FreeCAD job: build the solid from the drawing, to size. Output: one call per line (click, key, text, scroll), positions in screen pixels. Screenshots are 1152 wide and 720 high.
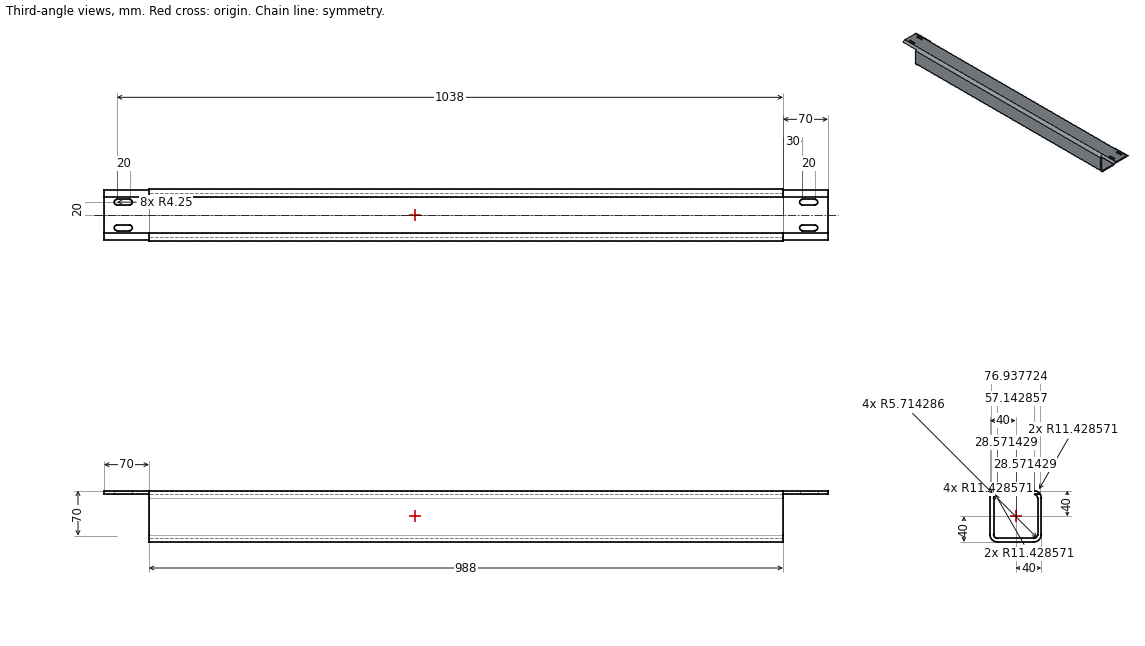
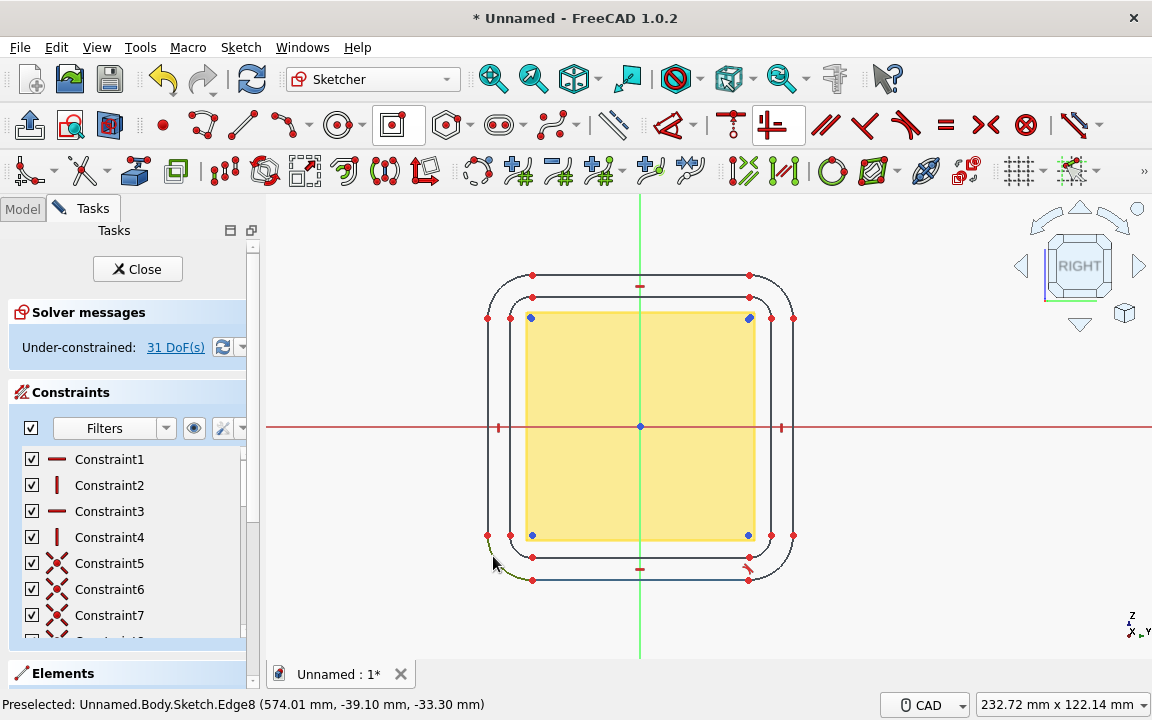
click(906, 126)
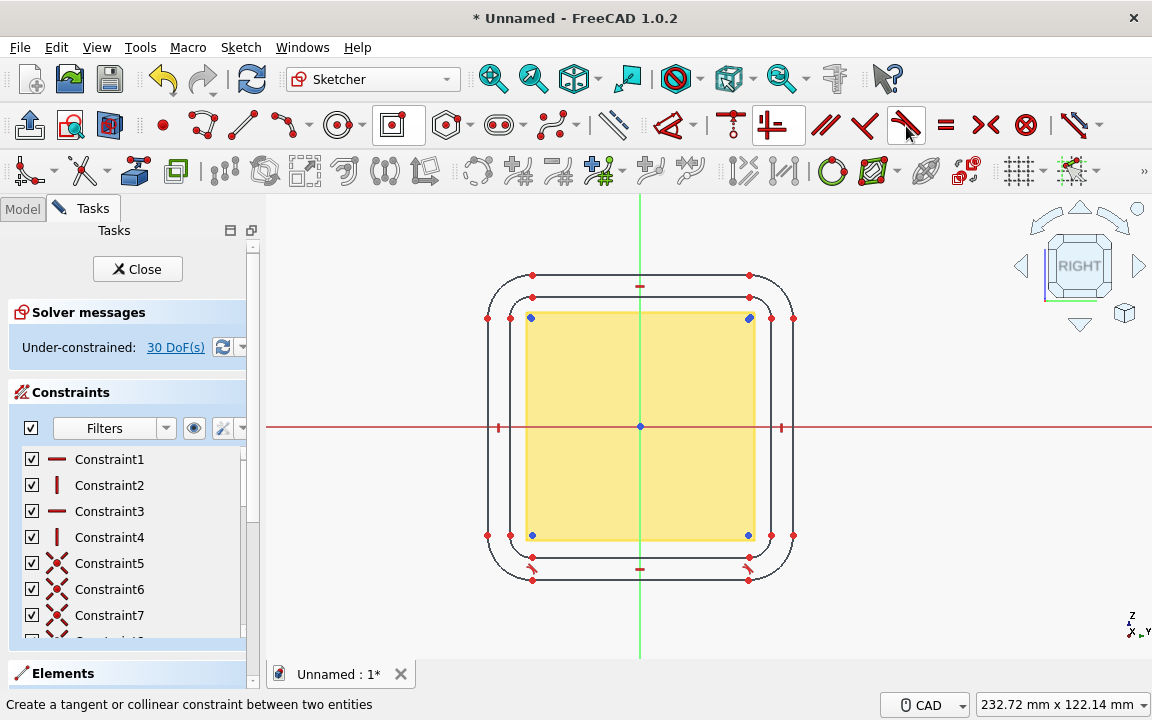
click(793, 471)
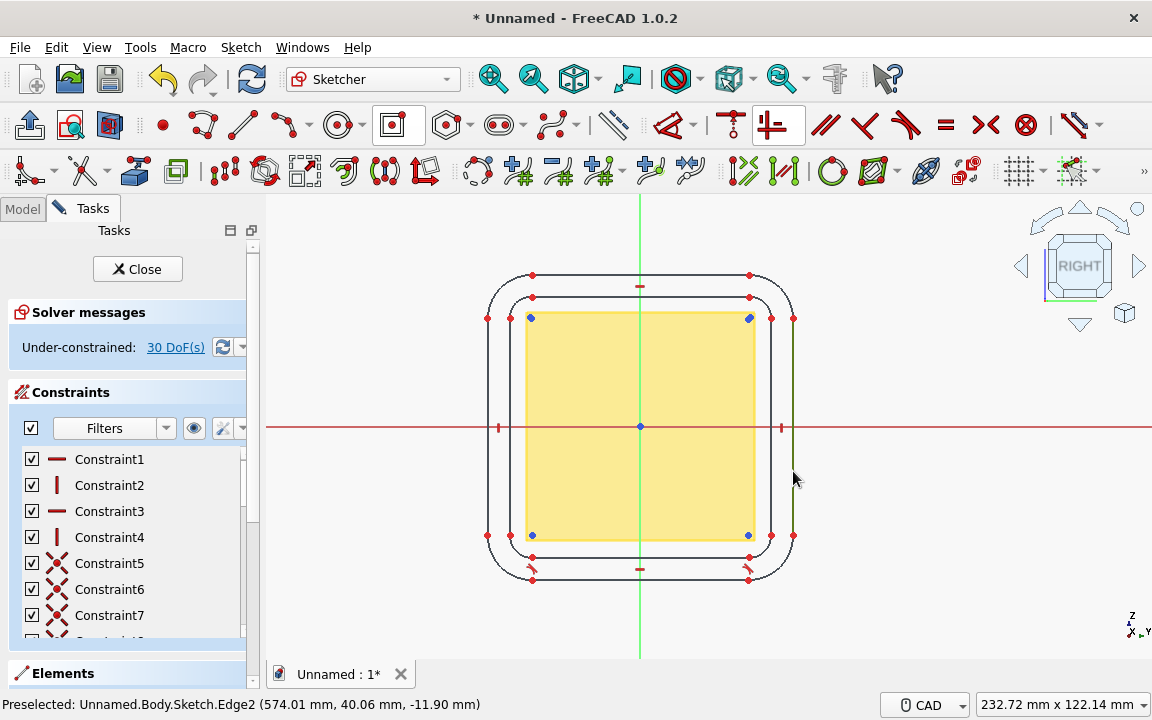
click(769, 575)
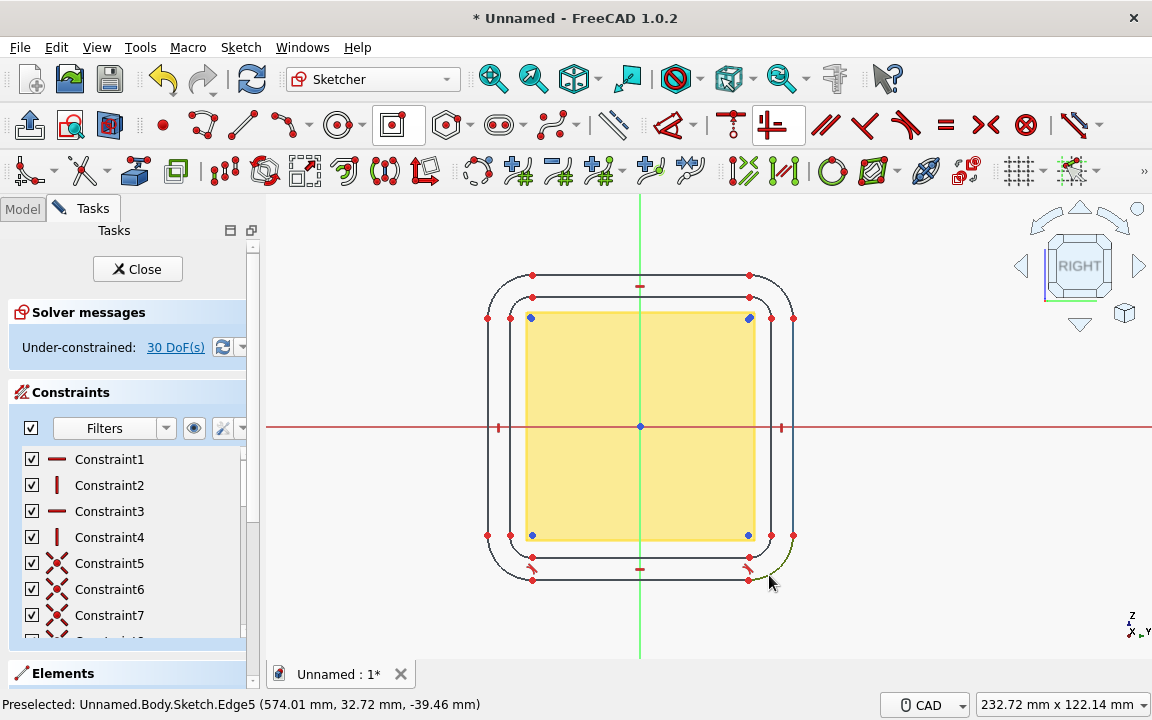
key(t)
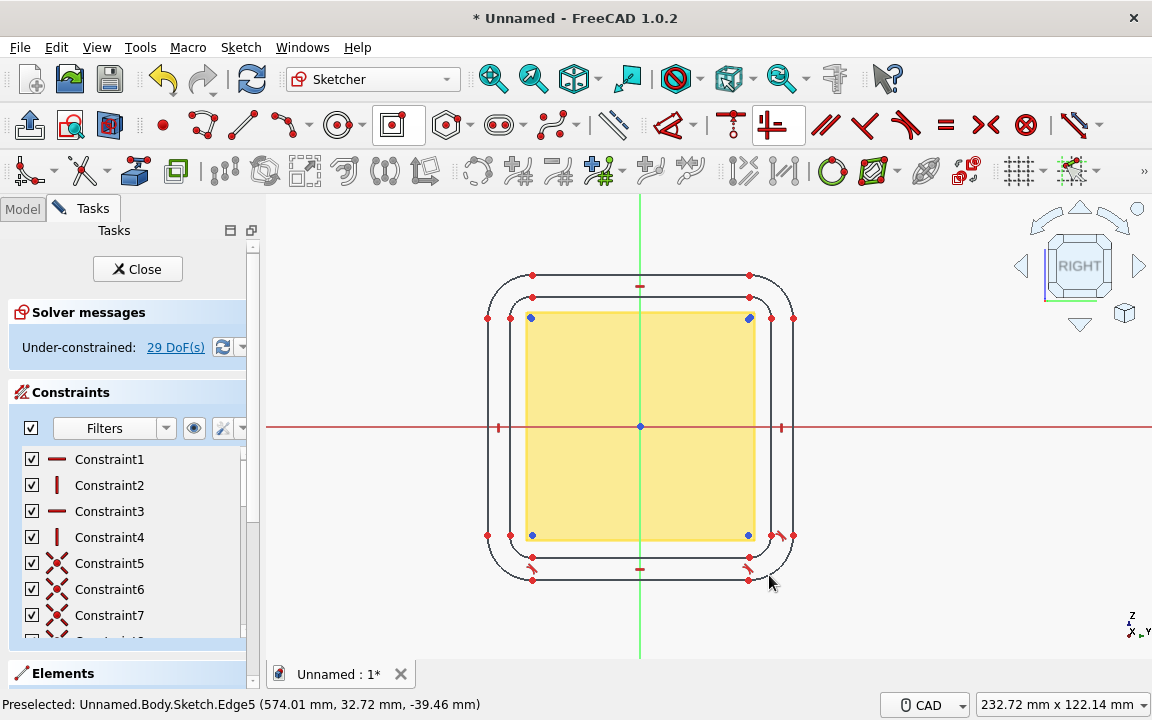
click(793, 471)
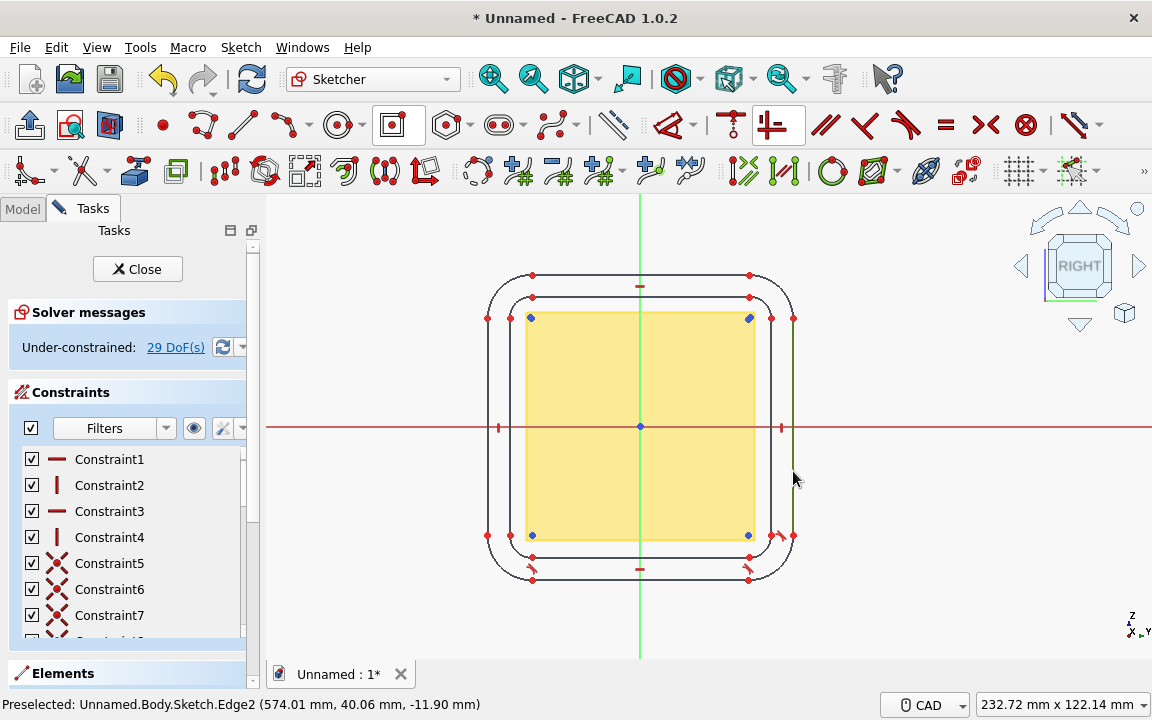
click(788, 299)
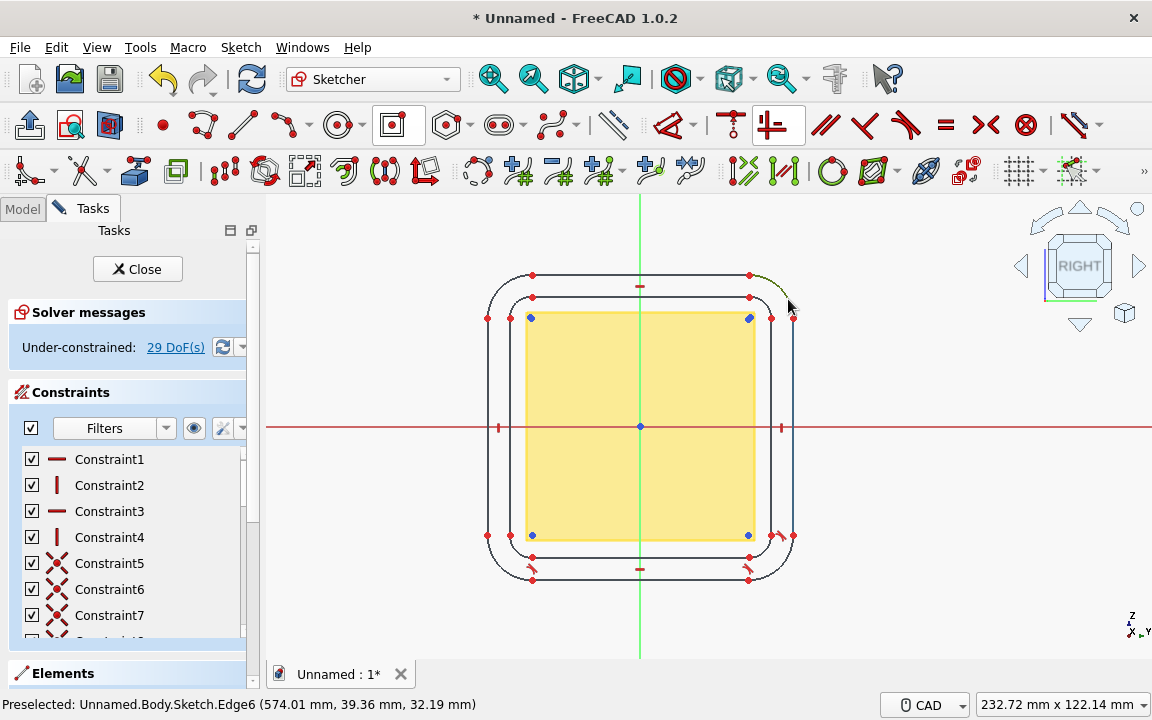
key(t)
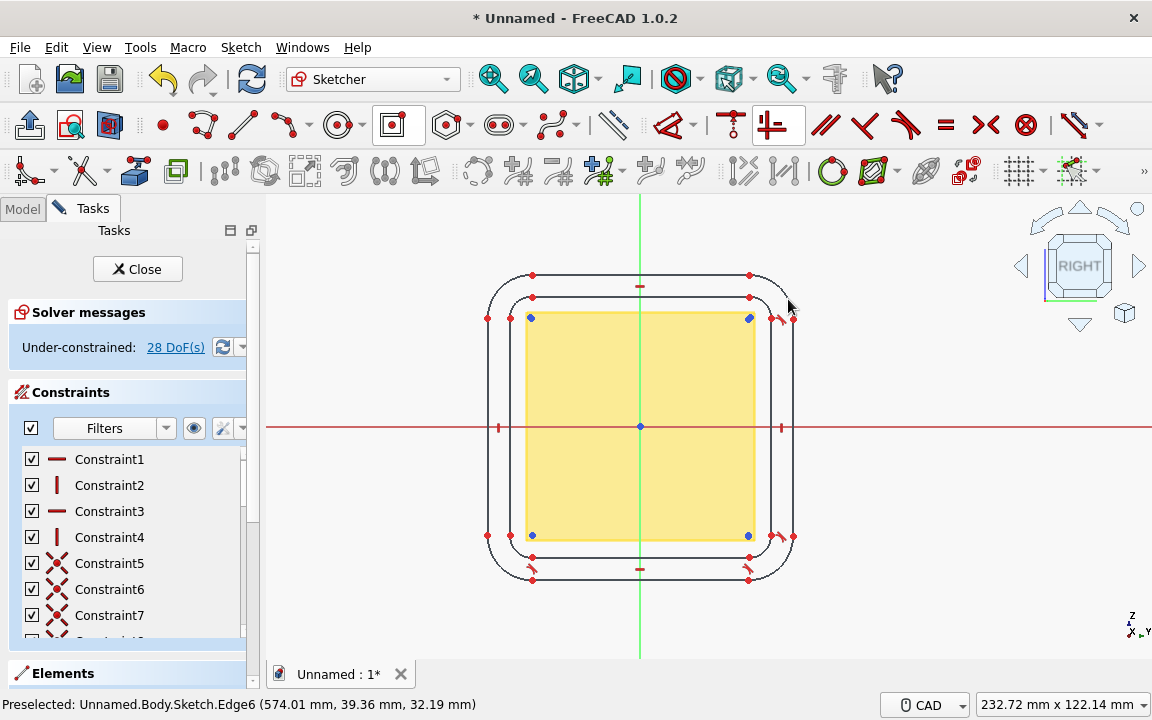
click(684, 275)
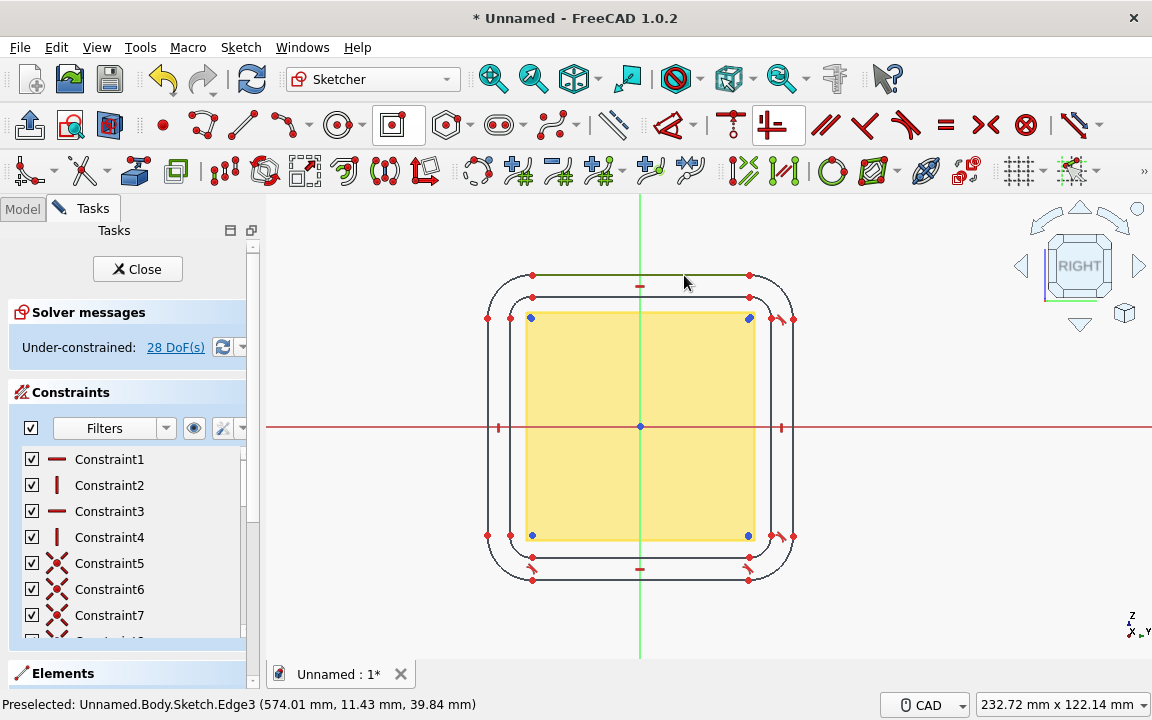
click(788, 299)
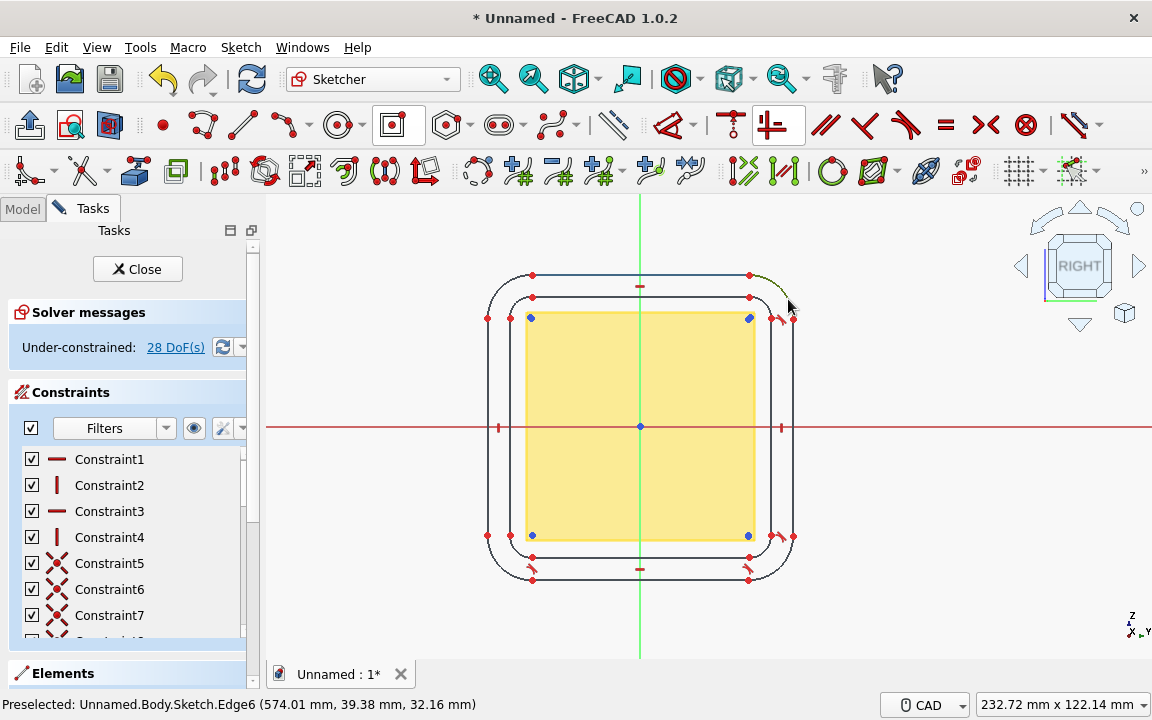
click(906, 126)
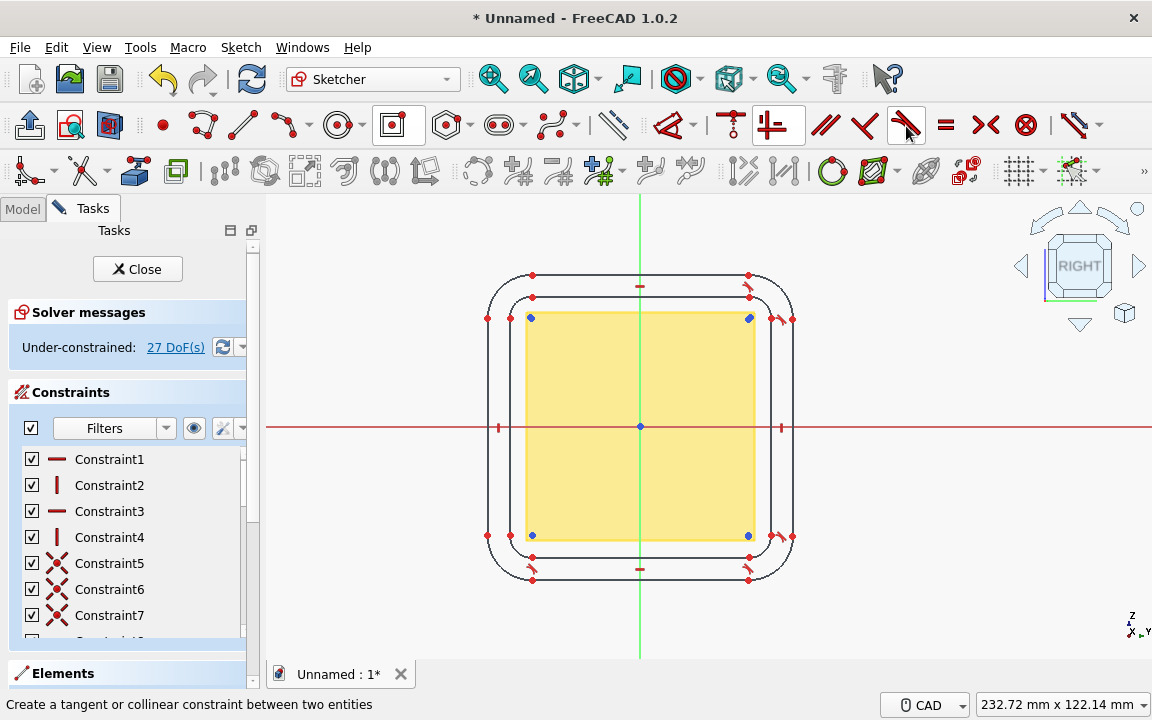
click(684, 275)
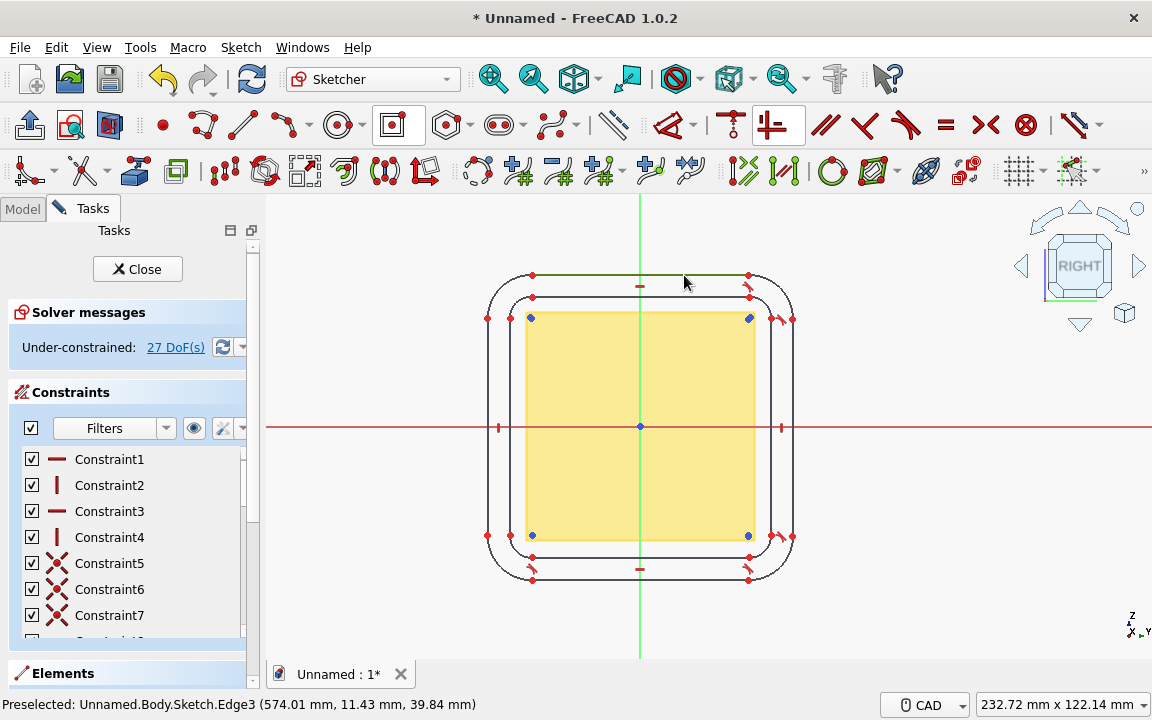
click(512, 280)